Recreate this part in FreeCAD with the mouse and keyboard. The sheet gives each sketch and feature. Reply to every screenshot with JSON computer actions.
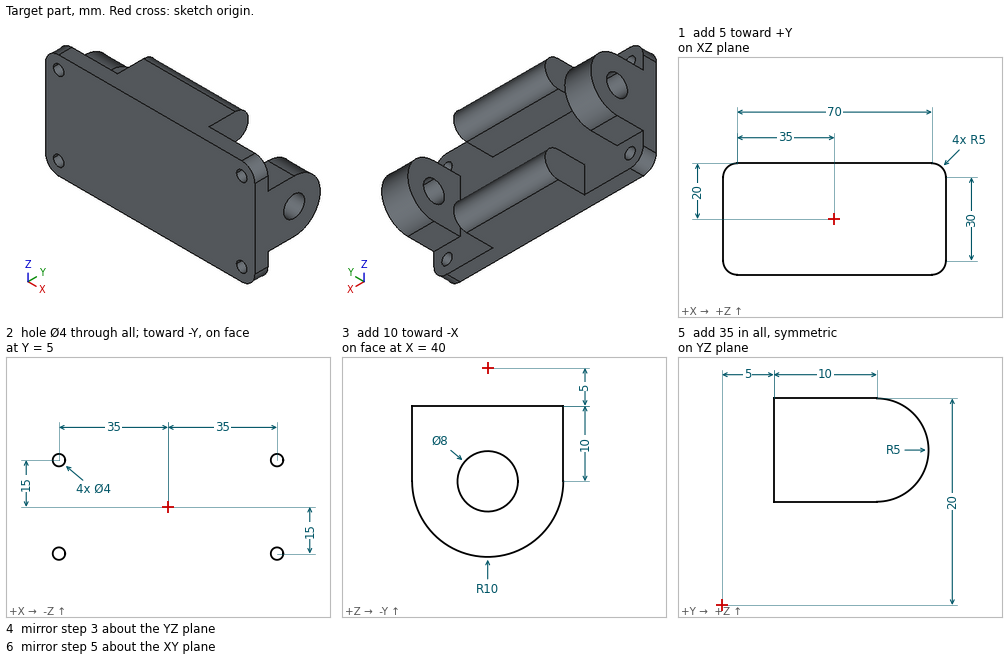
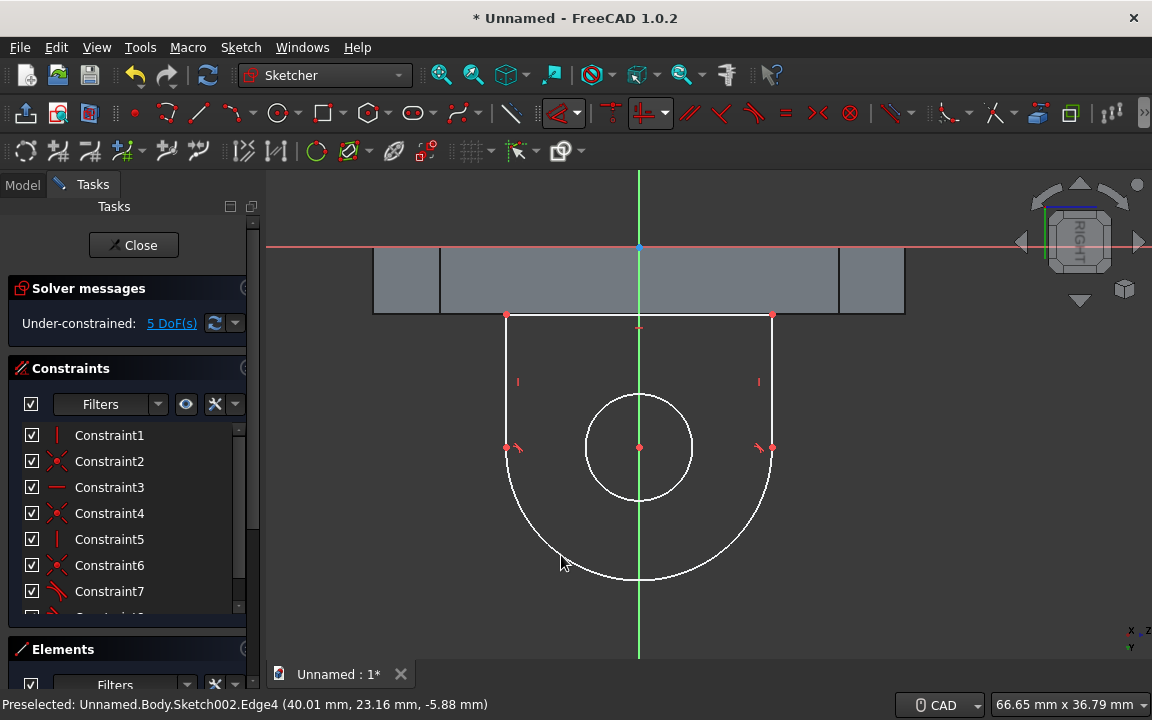
{"action": "left_click", "coordinate": [639, 447]}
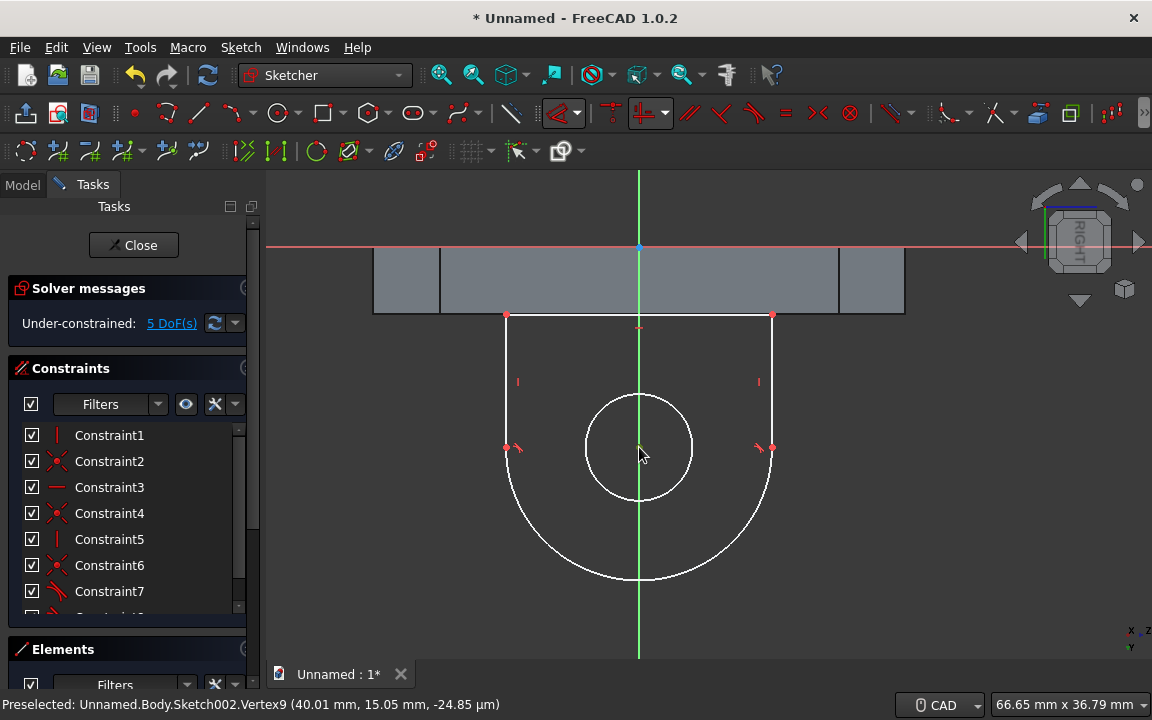
{"action": "left_click", "coordinate": [639, 538]}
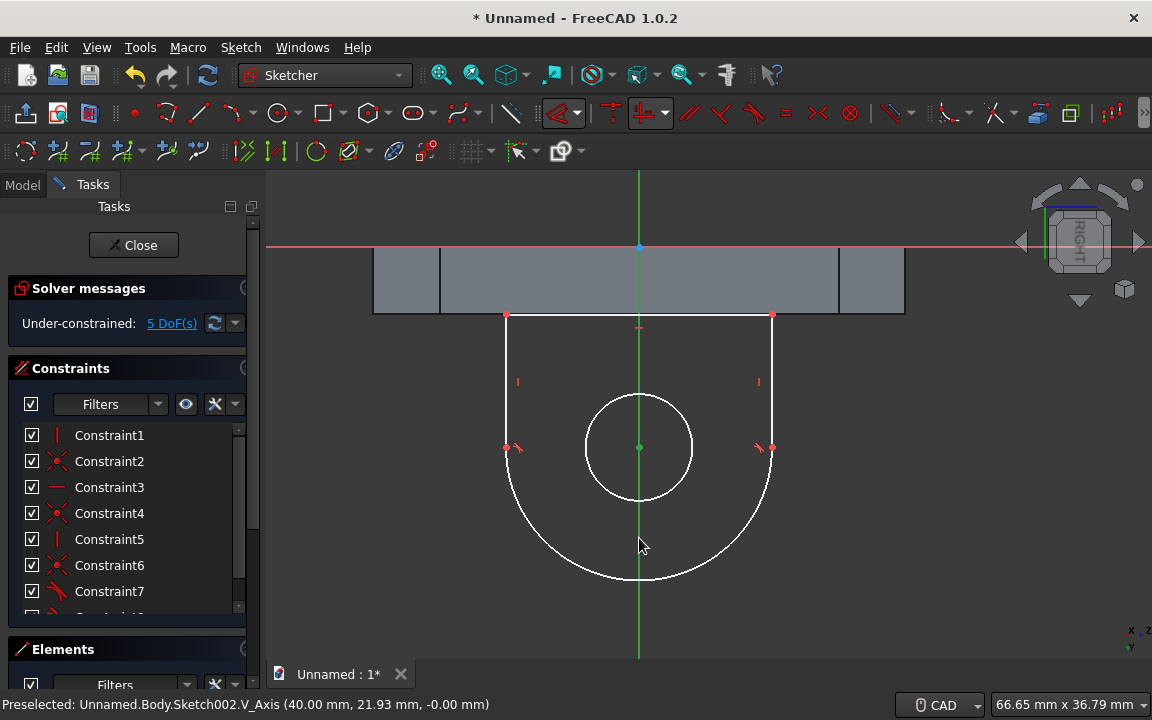
{"action": "key", "text": "c"}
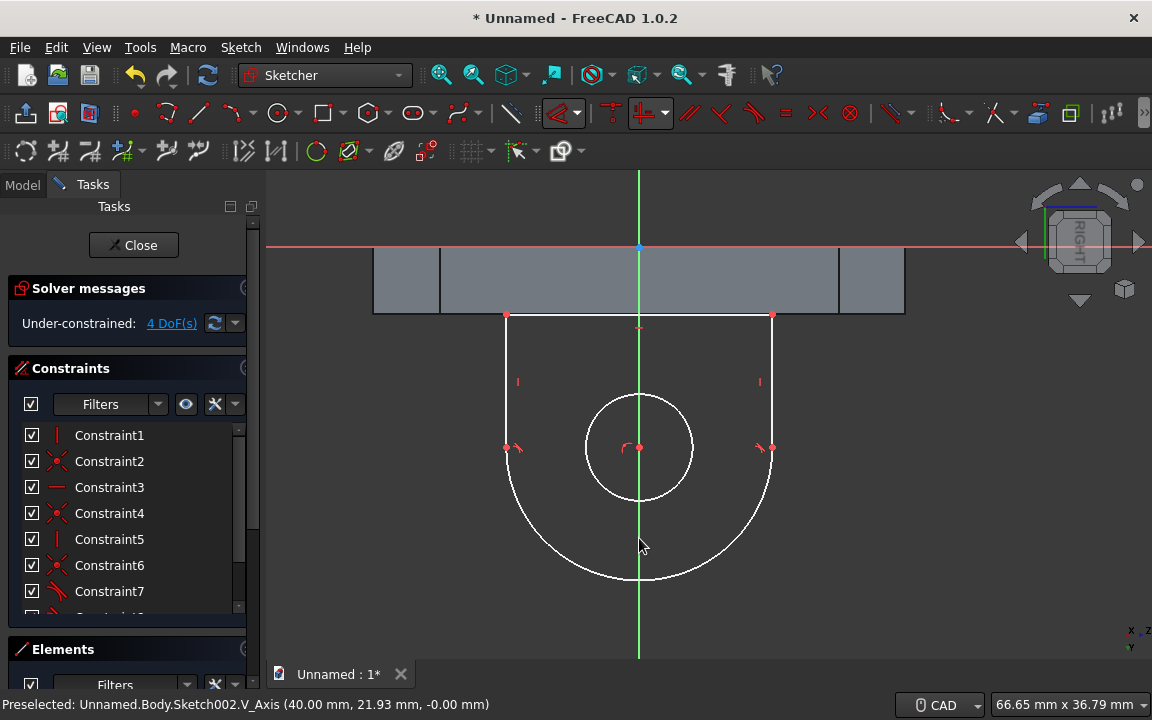
{"action": "left_click", "coordinate": [561, 555]}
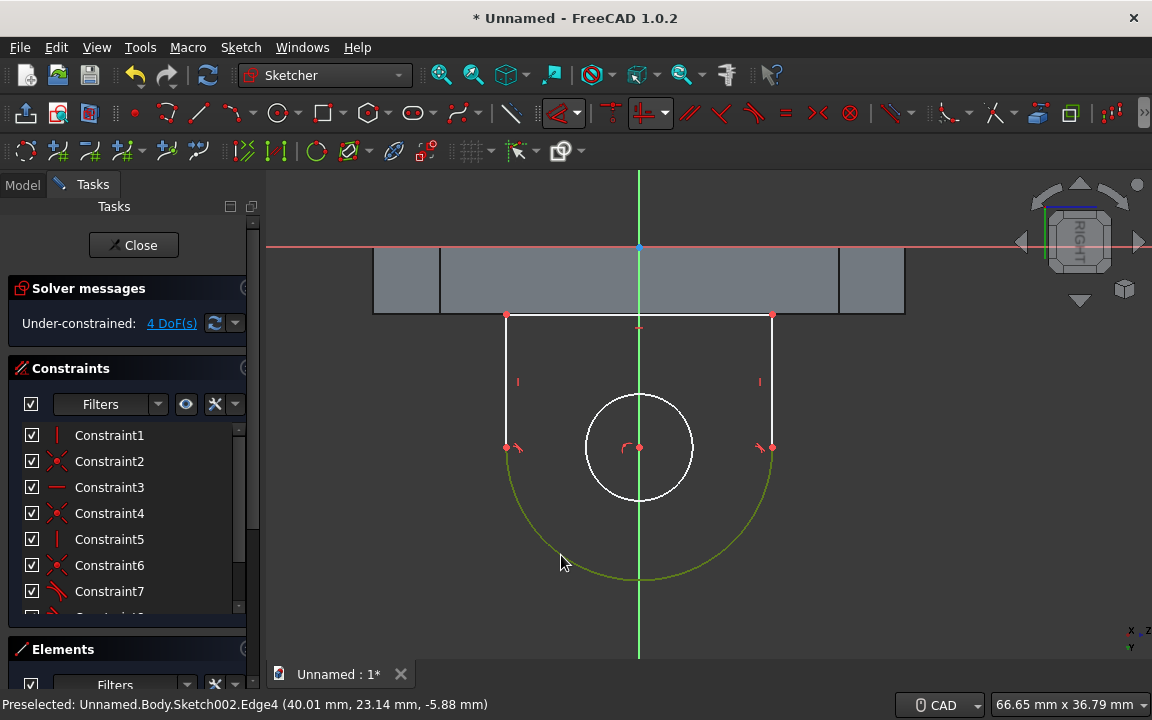
{"action": "key", "text": "k r"}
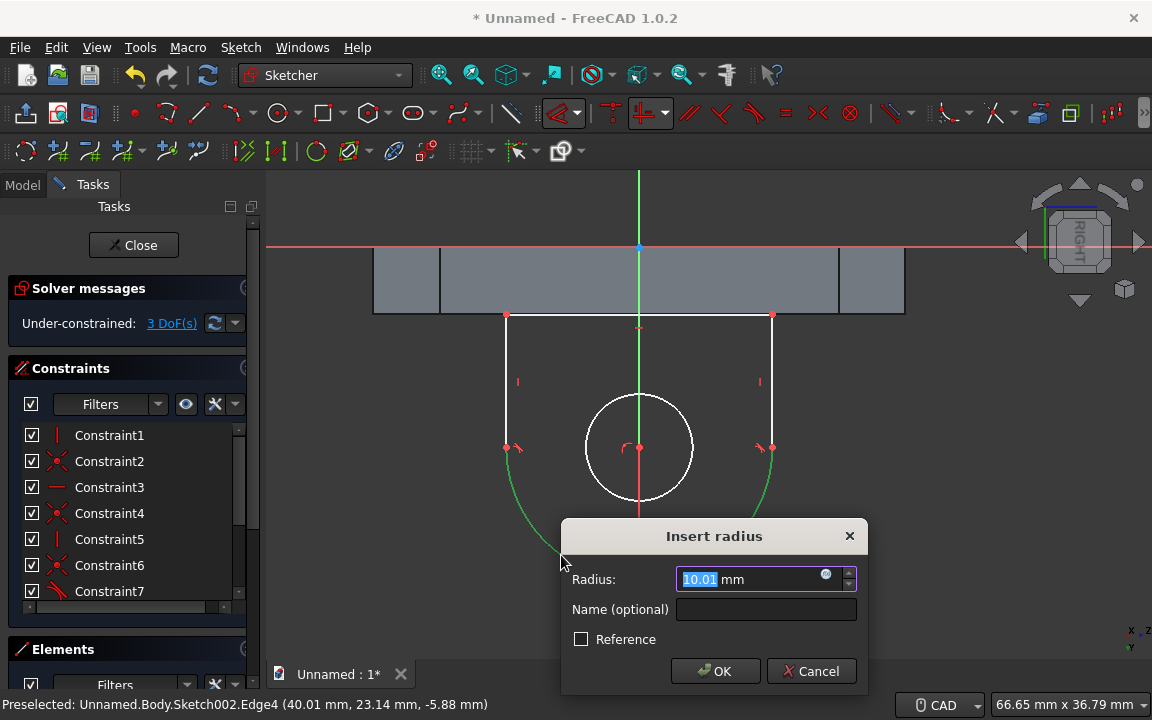
{"action": "type", "text": "10"}
{"action": "key", "text": "Return"}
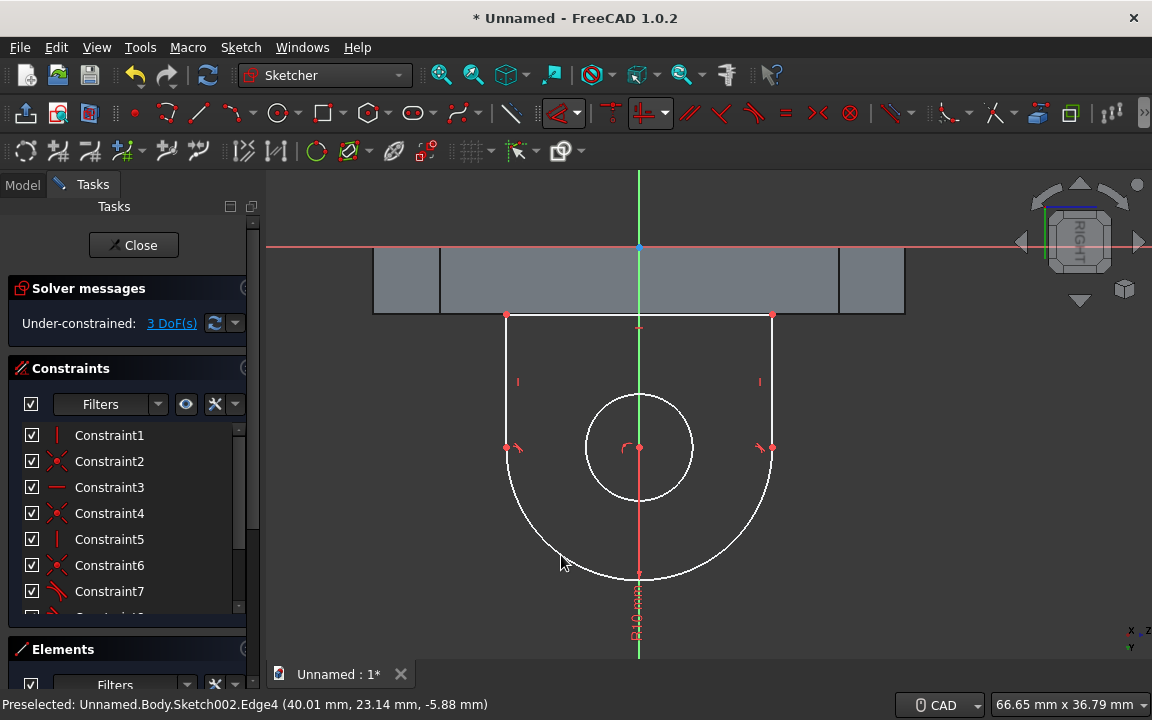
{"action": "left_click", "coordinate": [677, 410]}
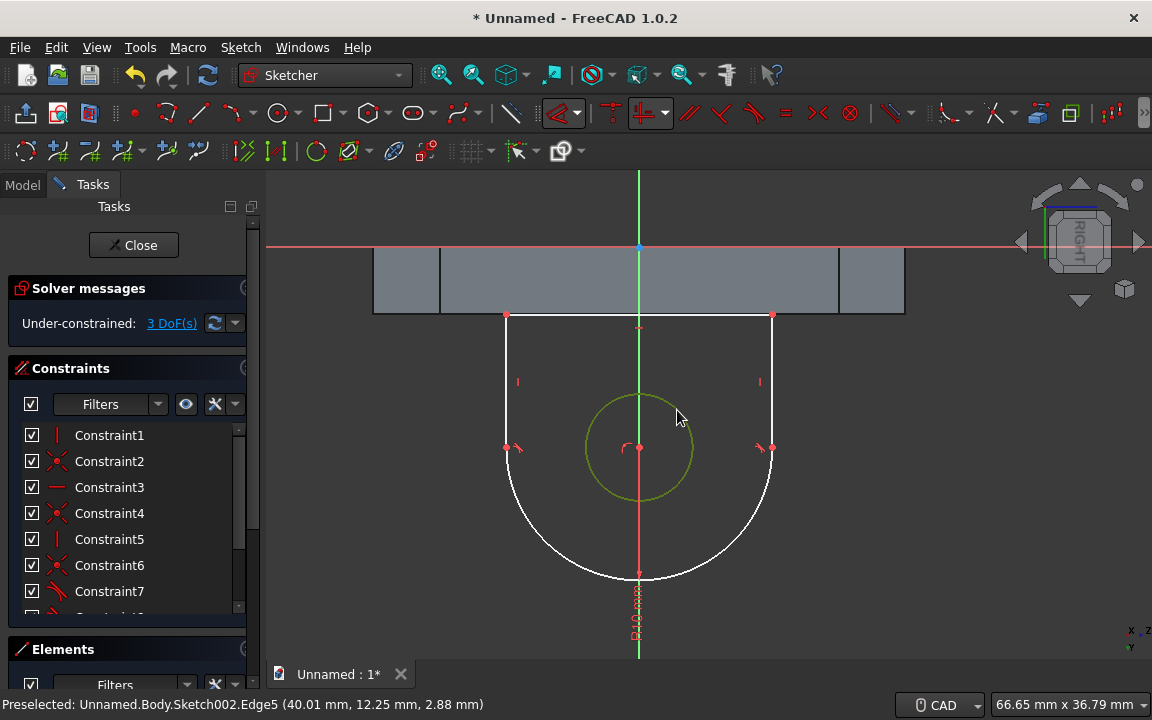
{"action": "key", "text": "k o"}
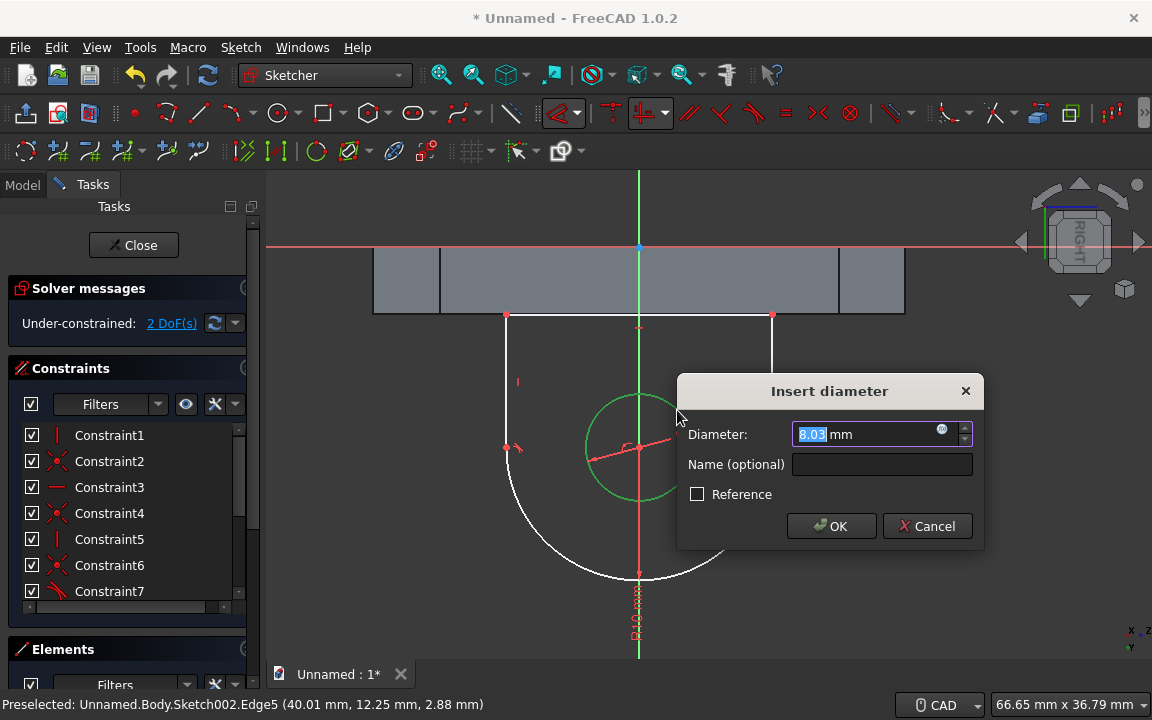
{"action": "type", "text": "8"}
{"action": "key", "text": "Return"}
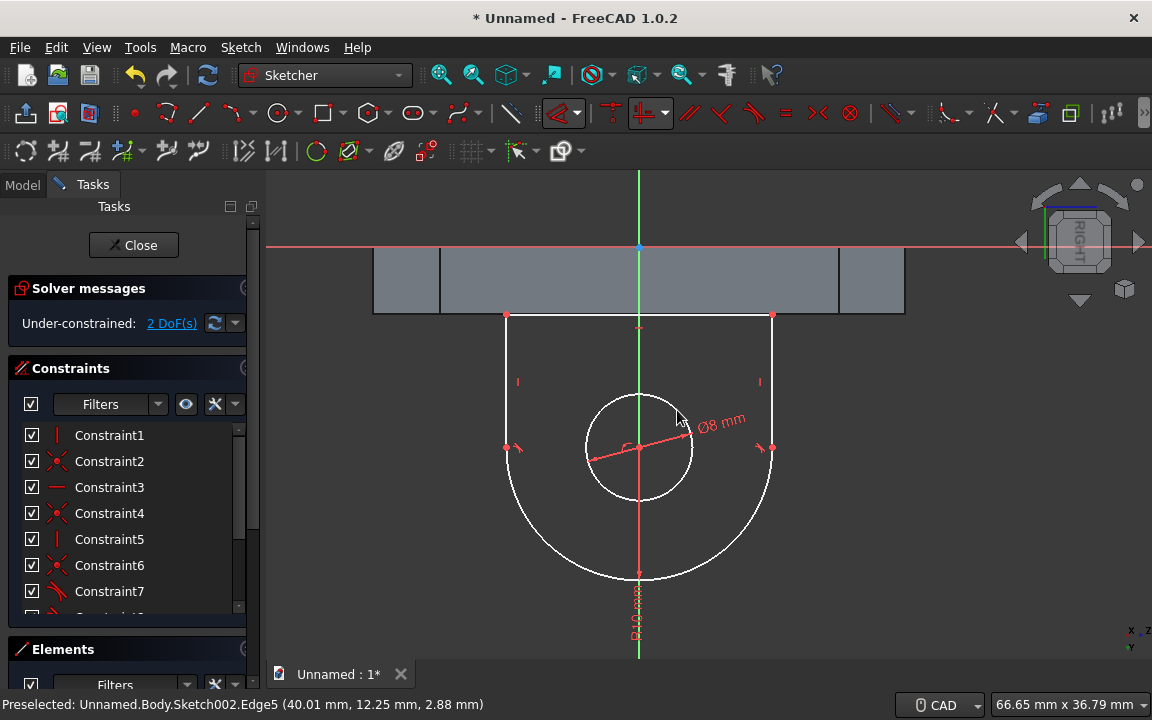
{"action": "left_click", "coordinate": [772, 408]}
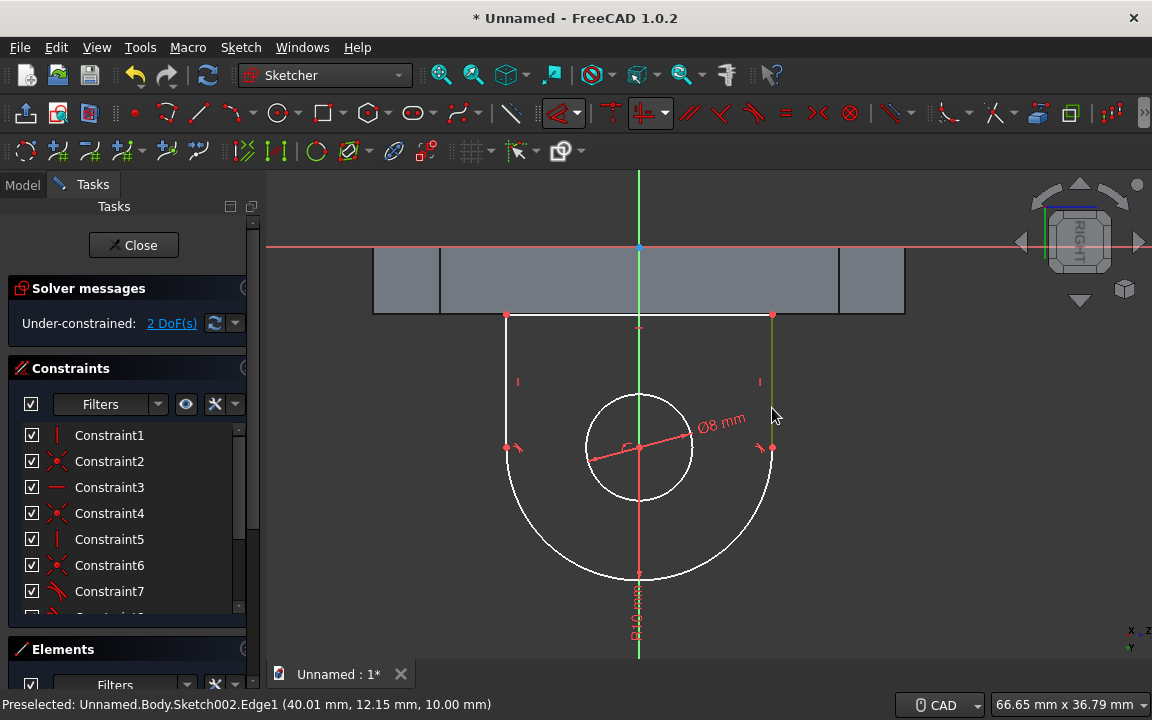
{"action": "key", "text": "i"}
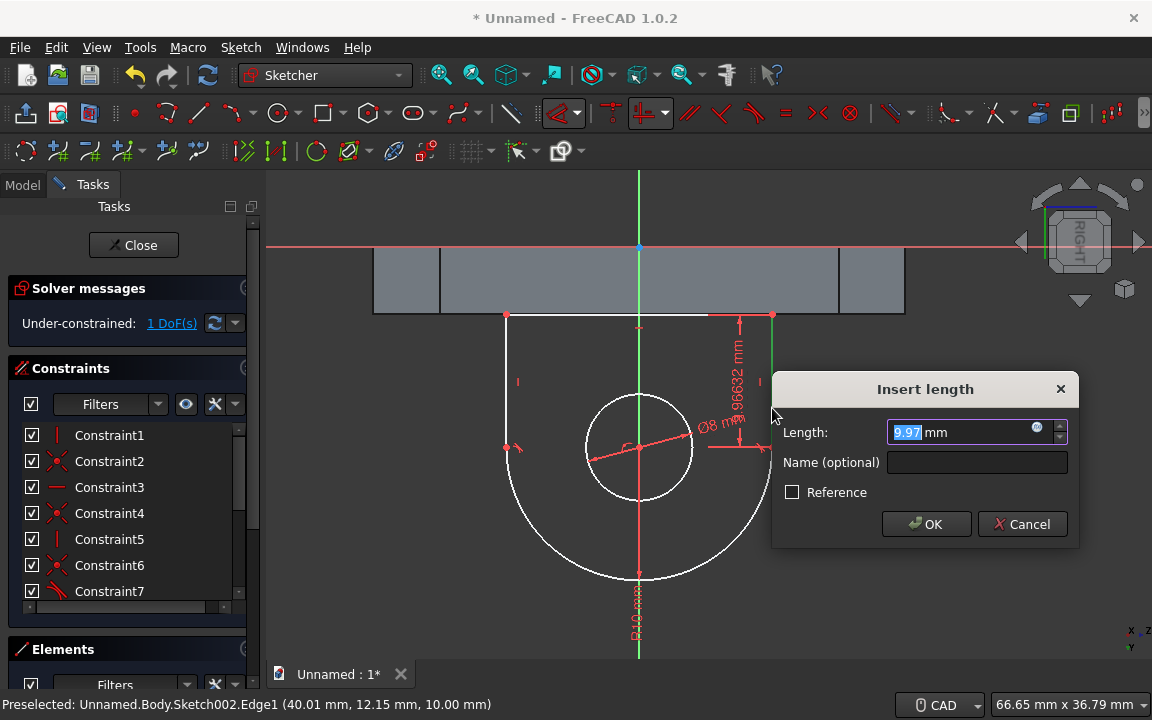
{"action": "type", "text": "10"}
{"action": "key", "text": "Return"}